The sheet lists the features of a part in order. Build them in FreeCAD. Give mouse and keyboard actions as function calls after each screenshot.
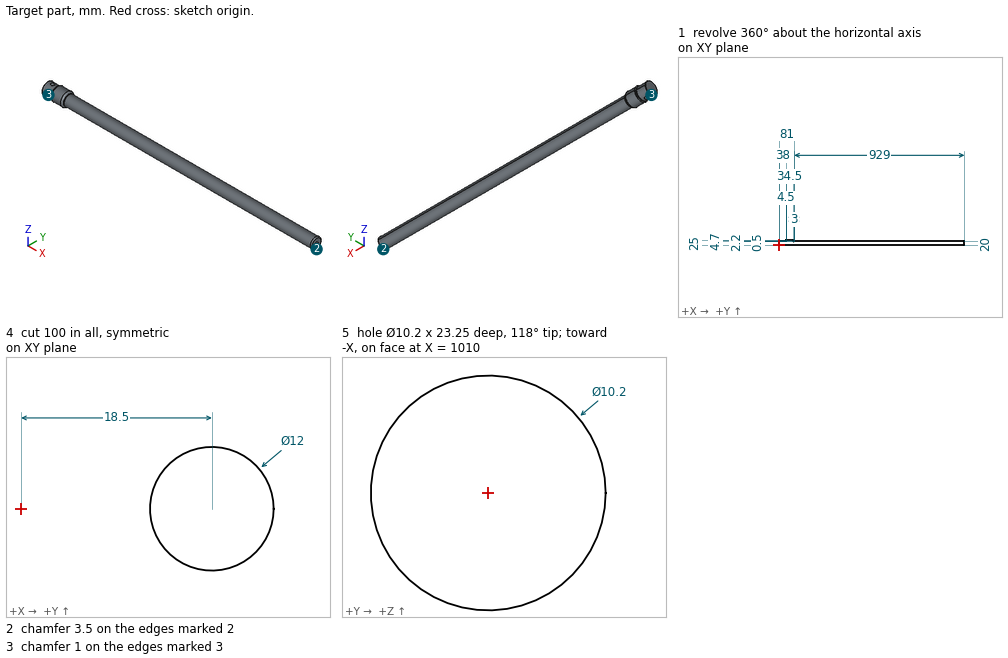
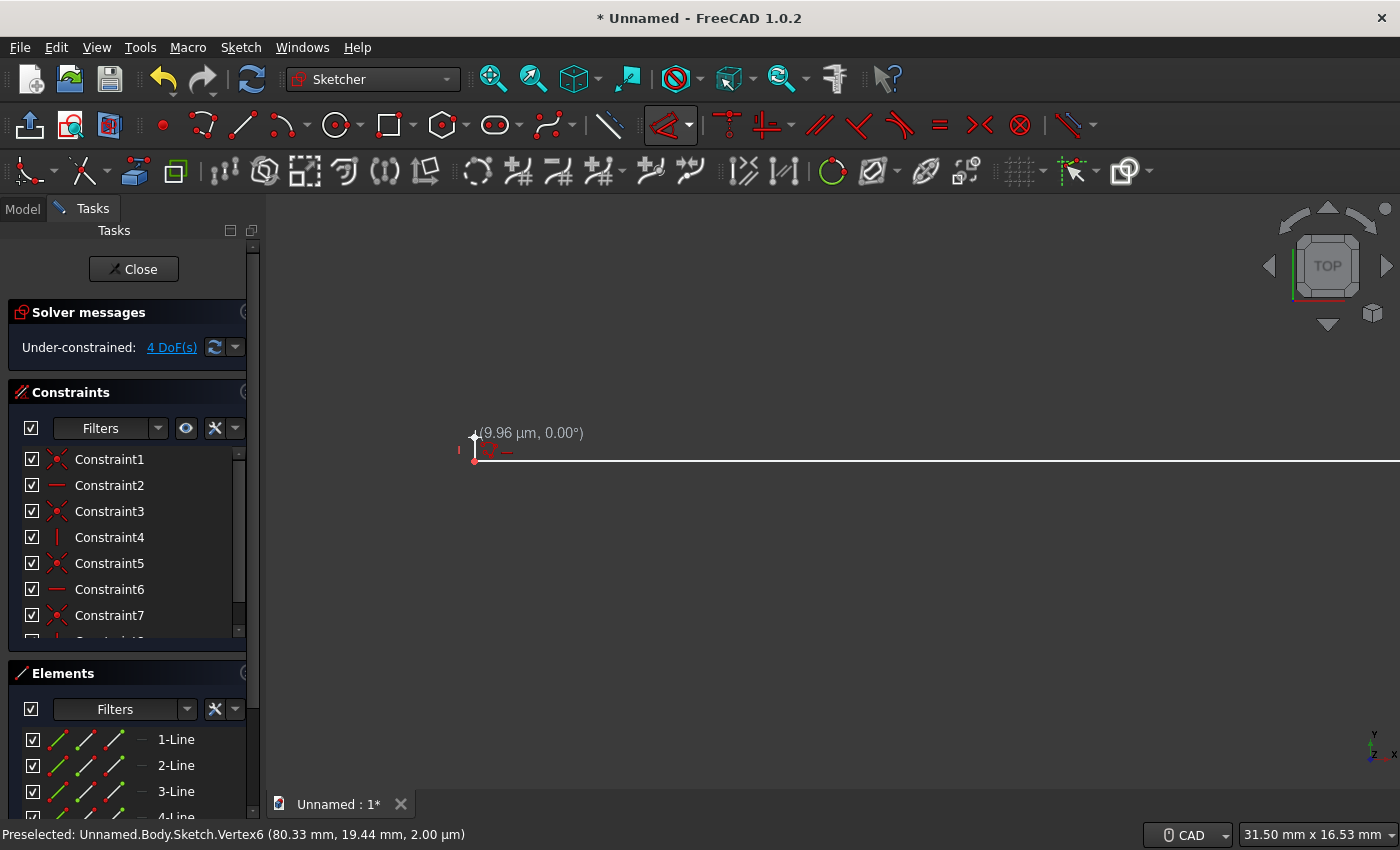
scroll(764, 492, down, 15)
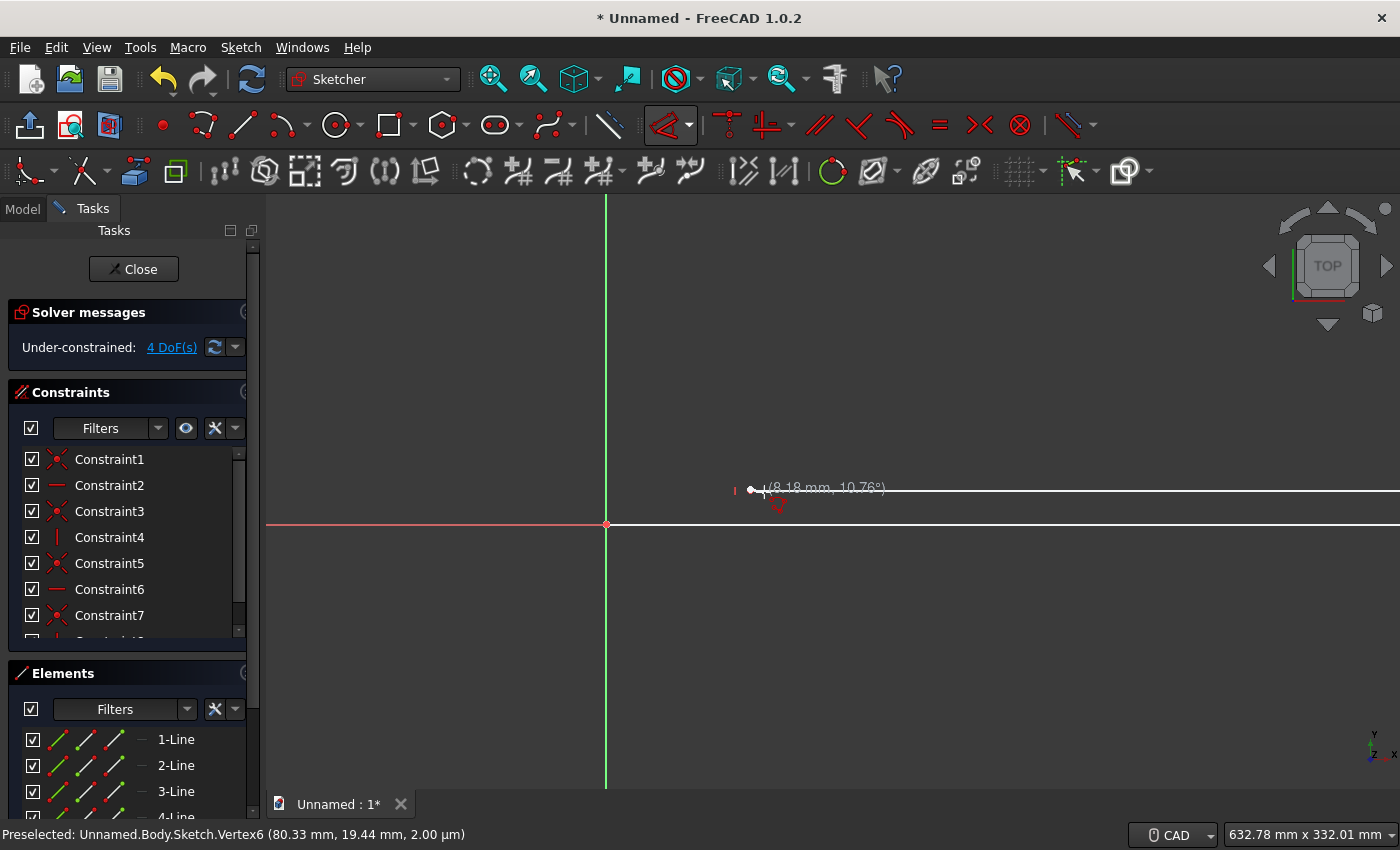
scroll(330, 485, down, 5)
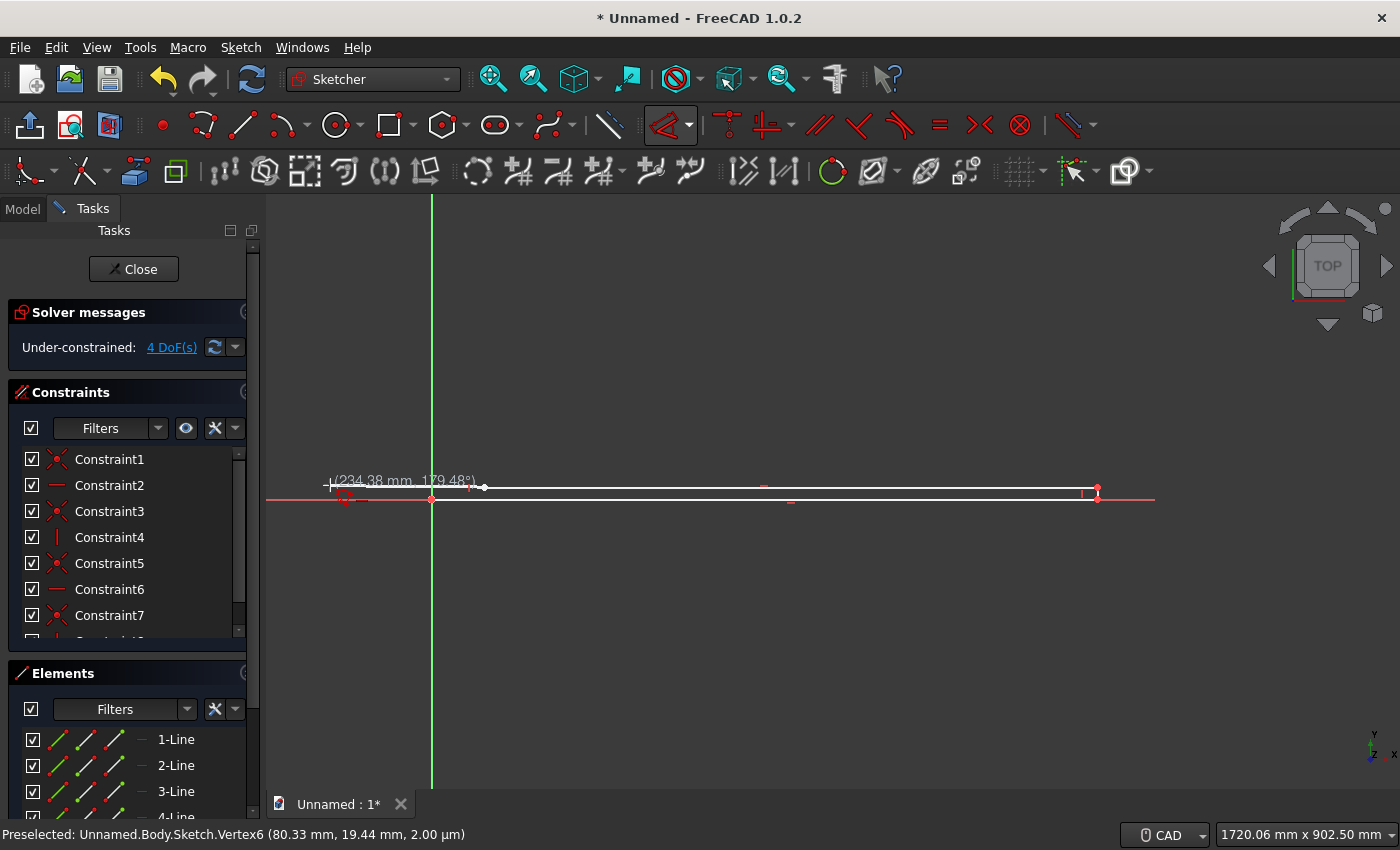
scroll(483, 487, up, 11)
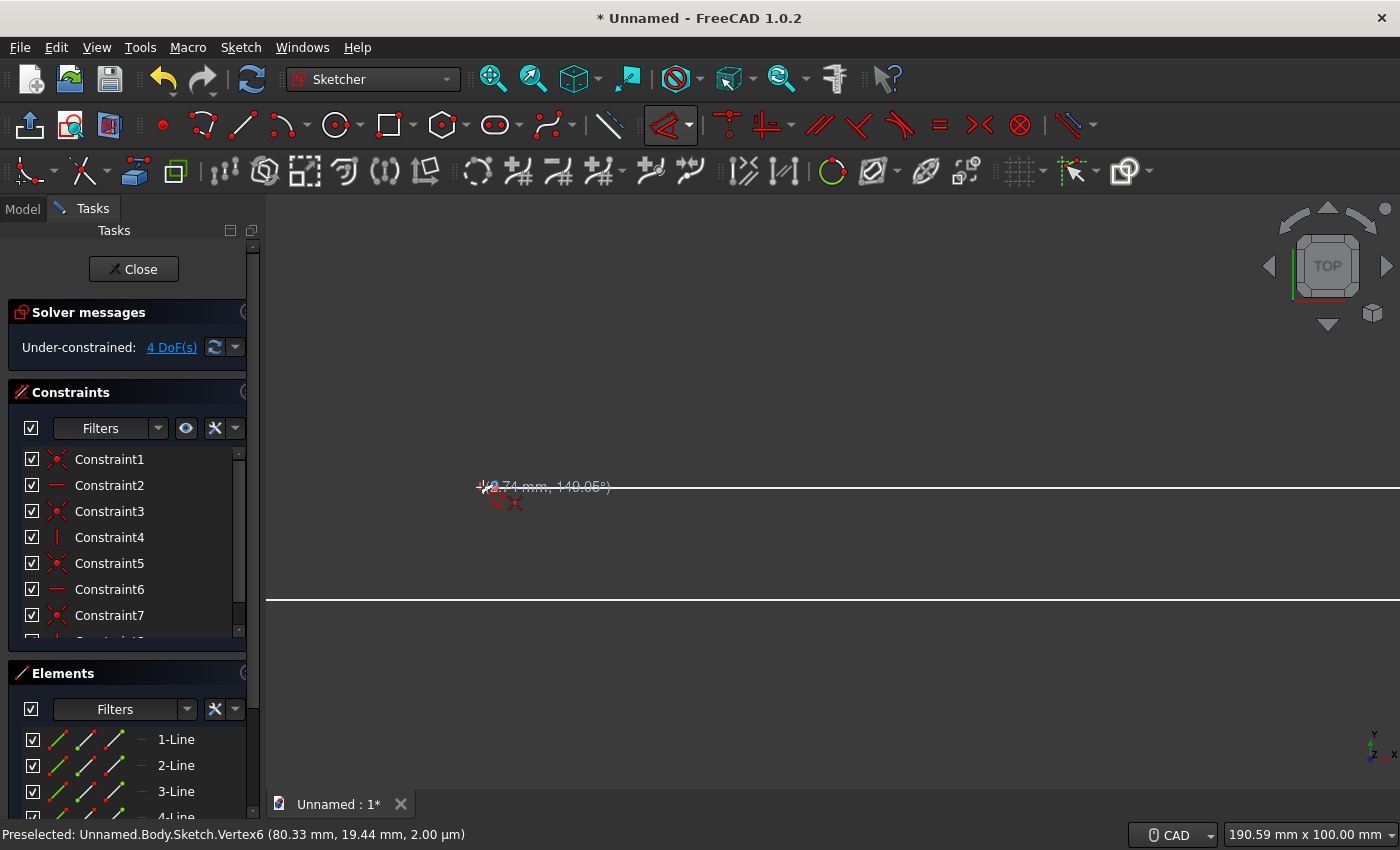
click(482, 484)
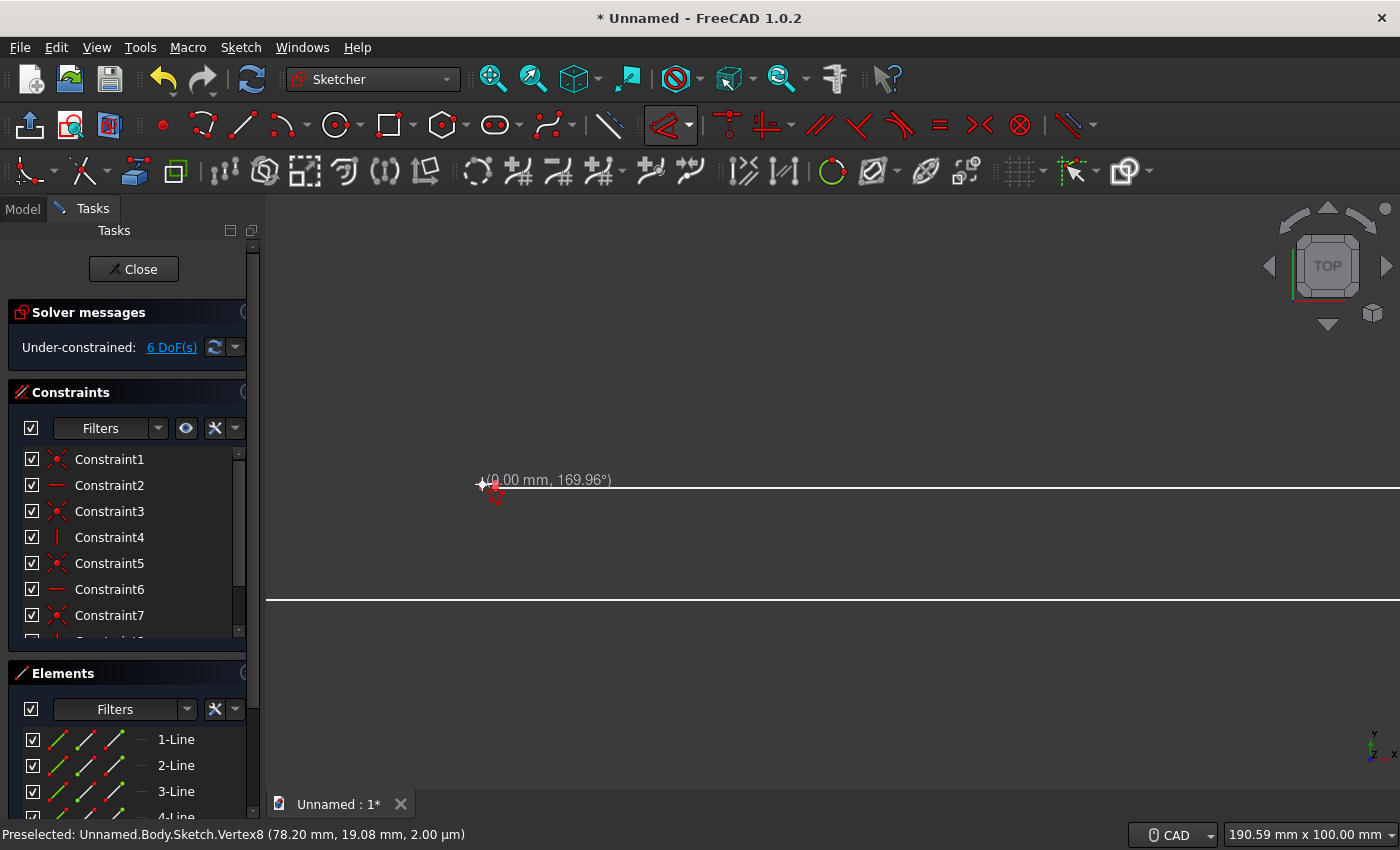
scroll(483, 487, down, 11)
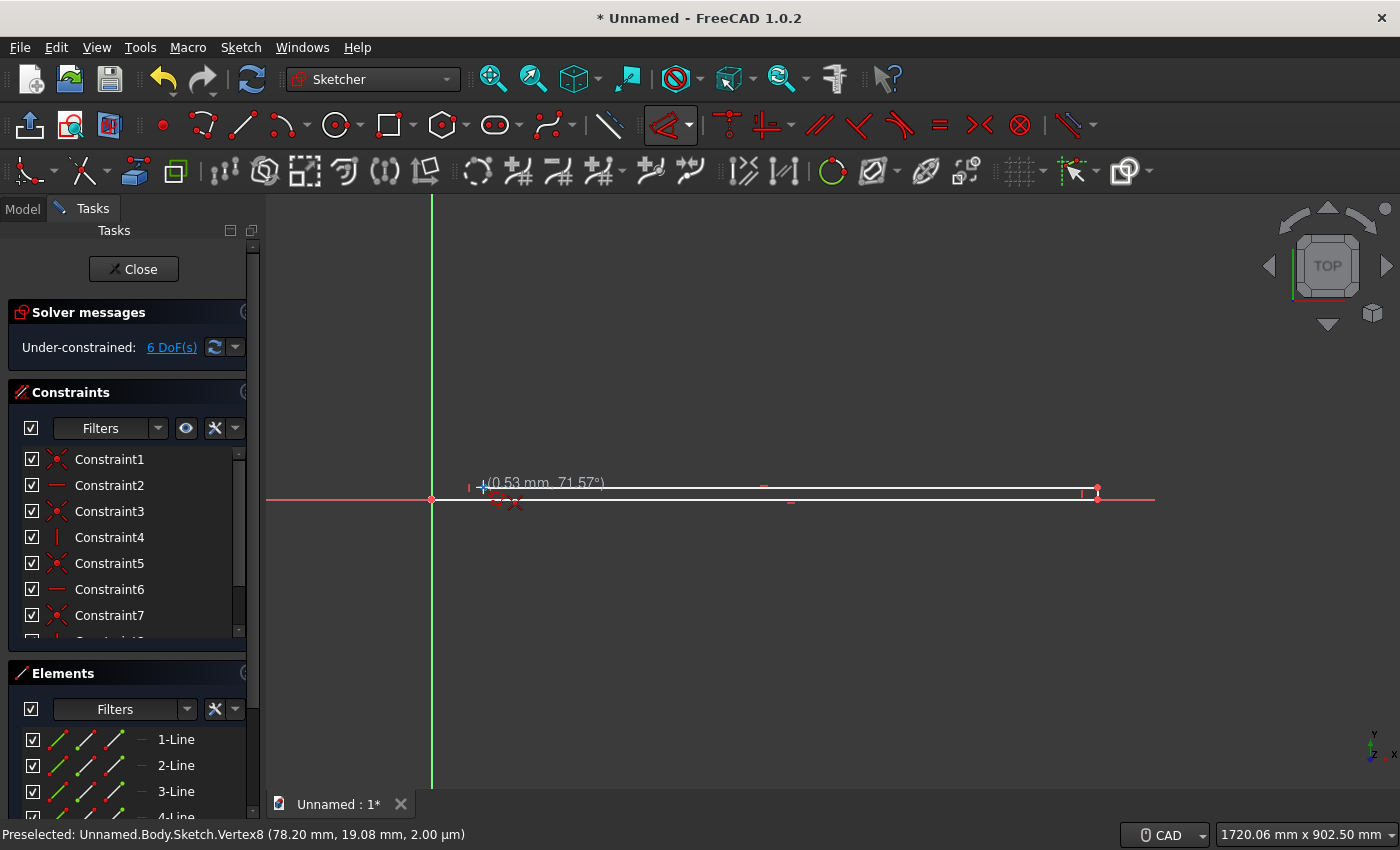
scroll(479, 483, up, 6)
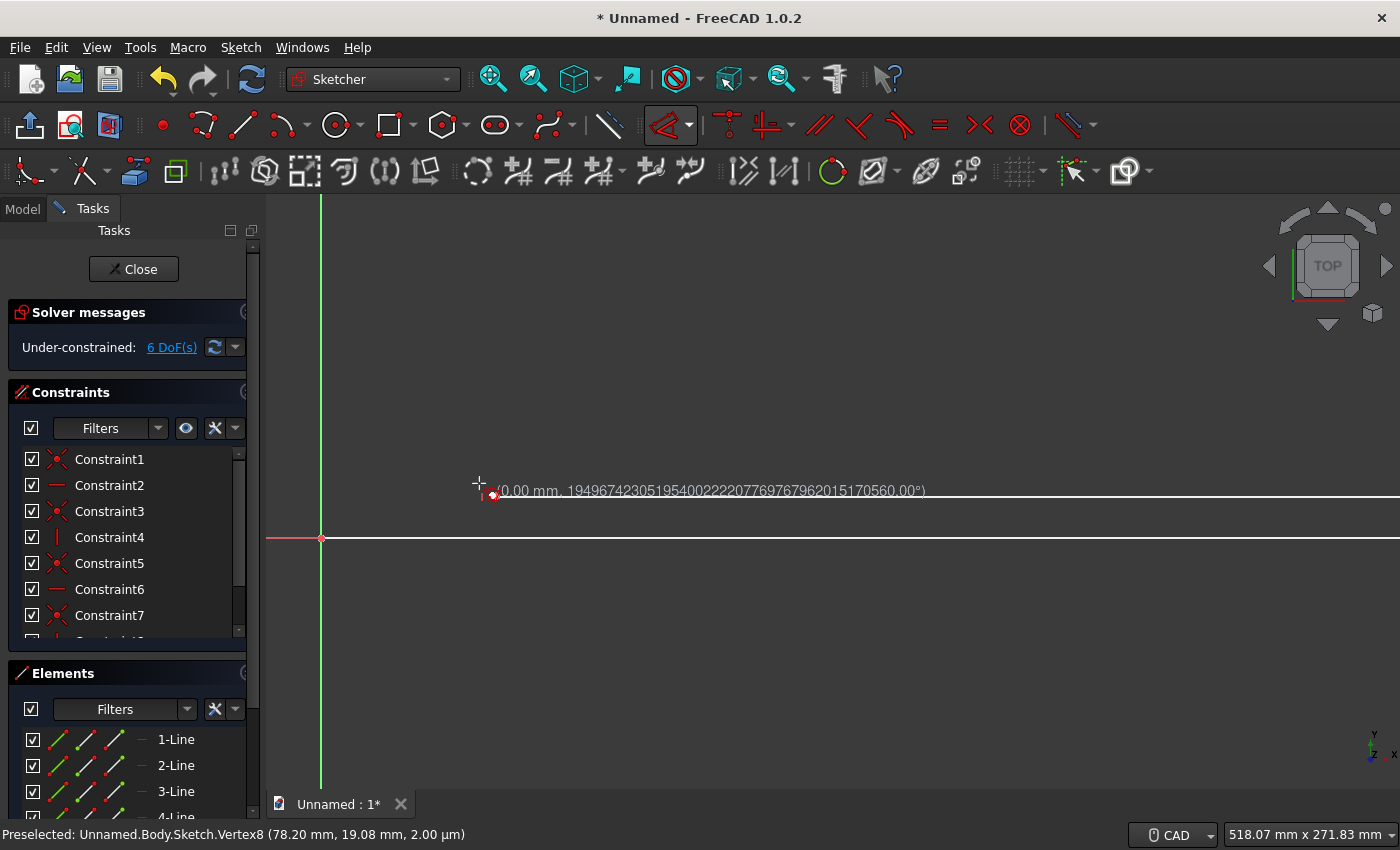
click(480, 483)
click(404, 483)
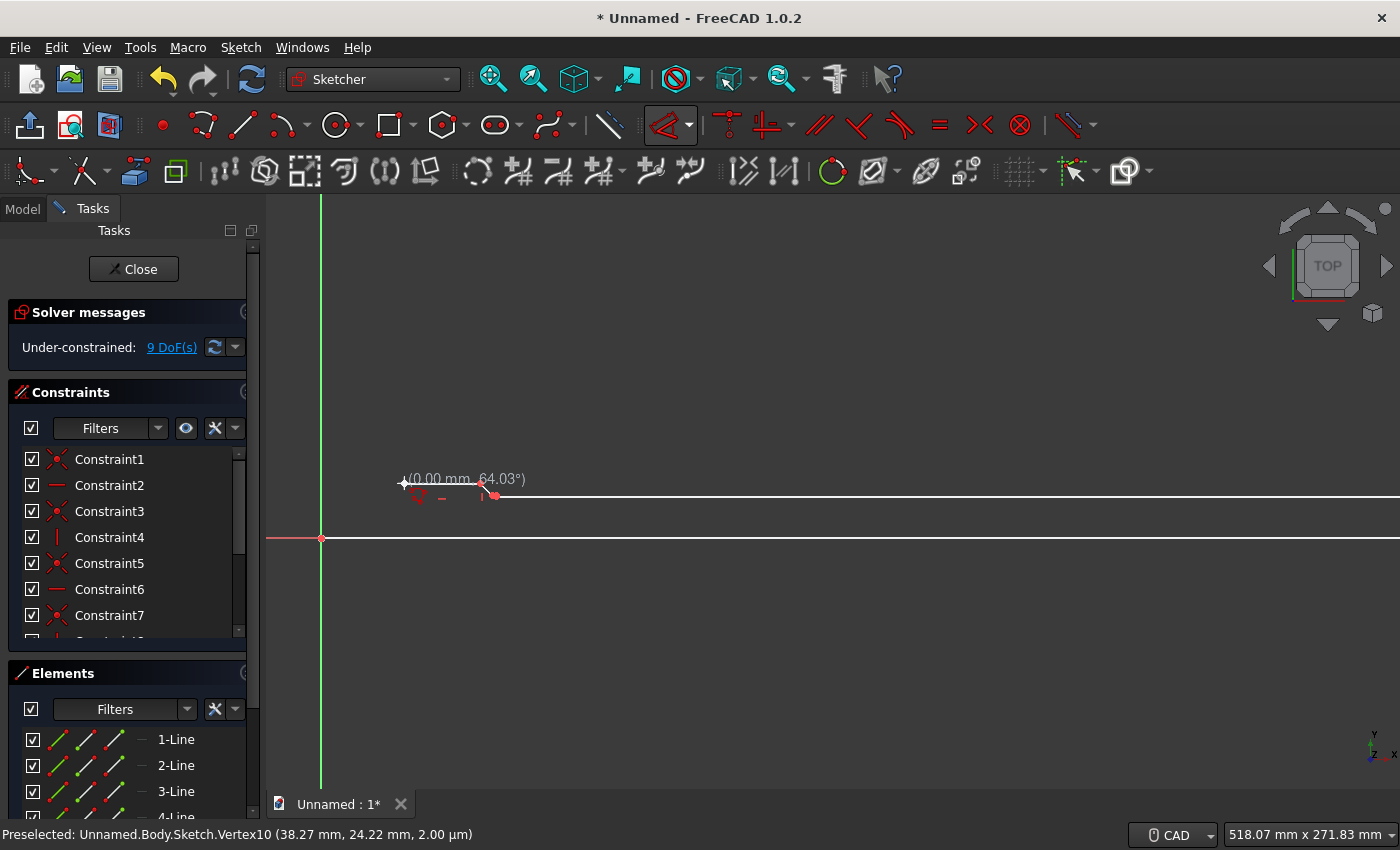
scroll(404, 494, up, 3)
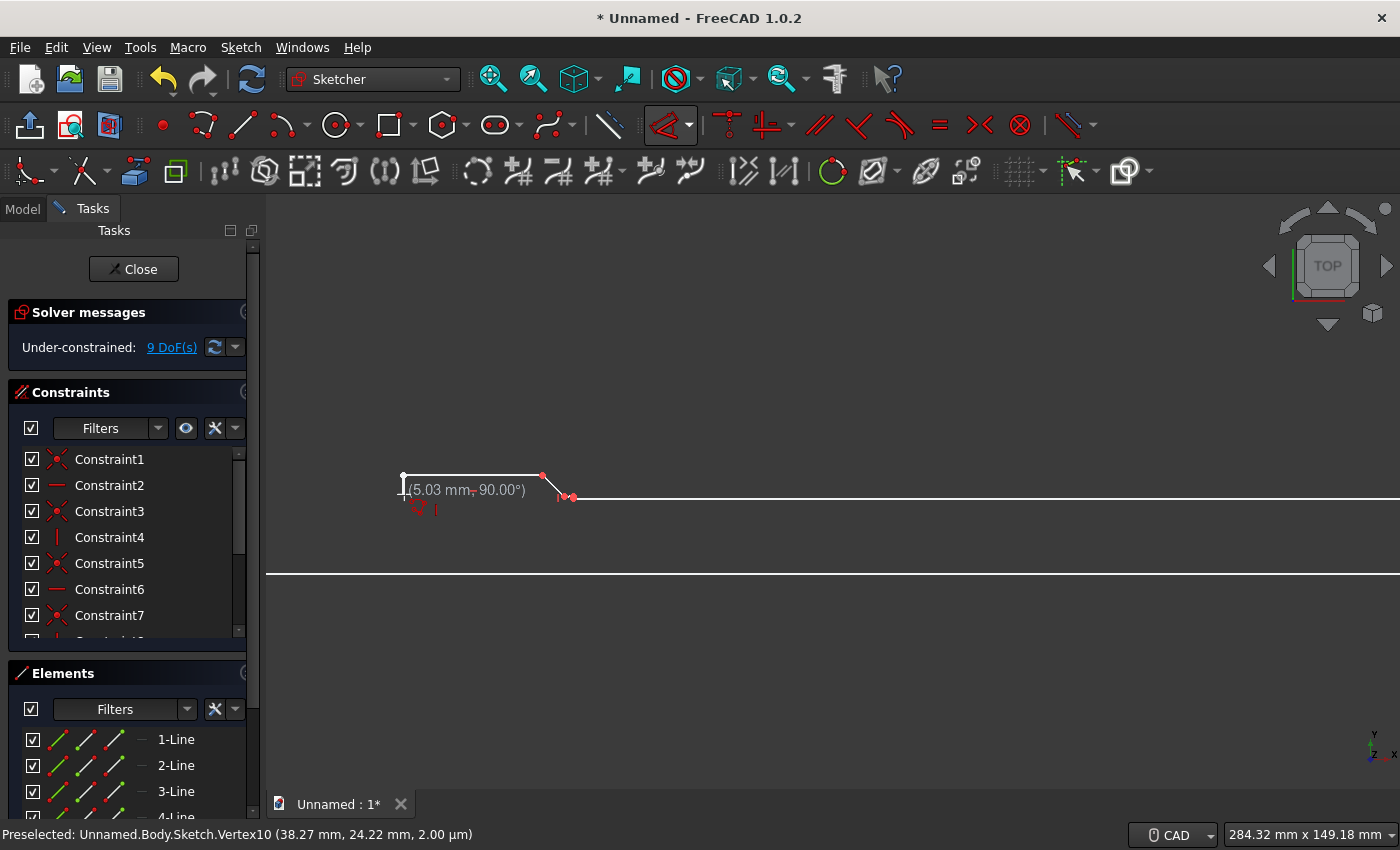
click(404, 493)
click(387, 493)